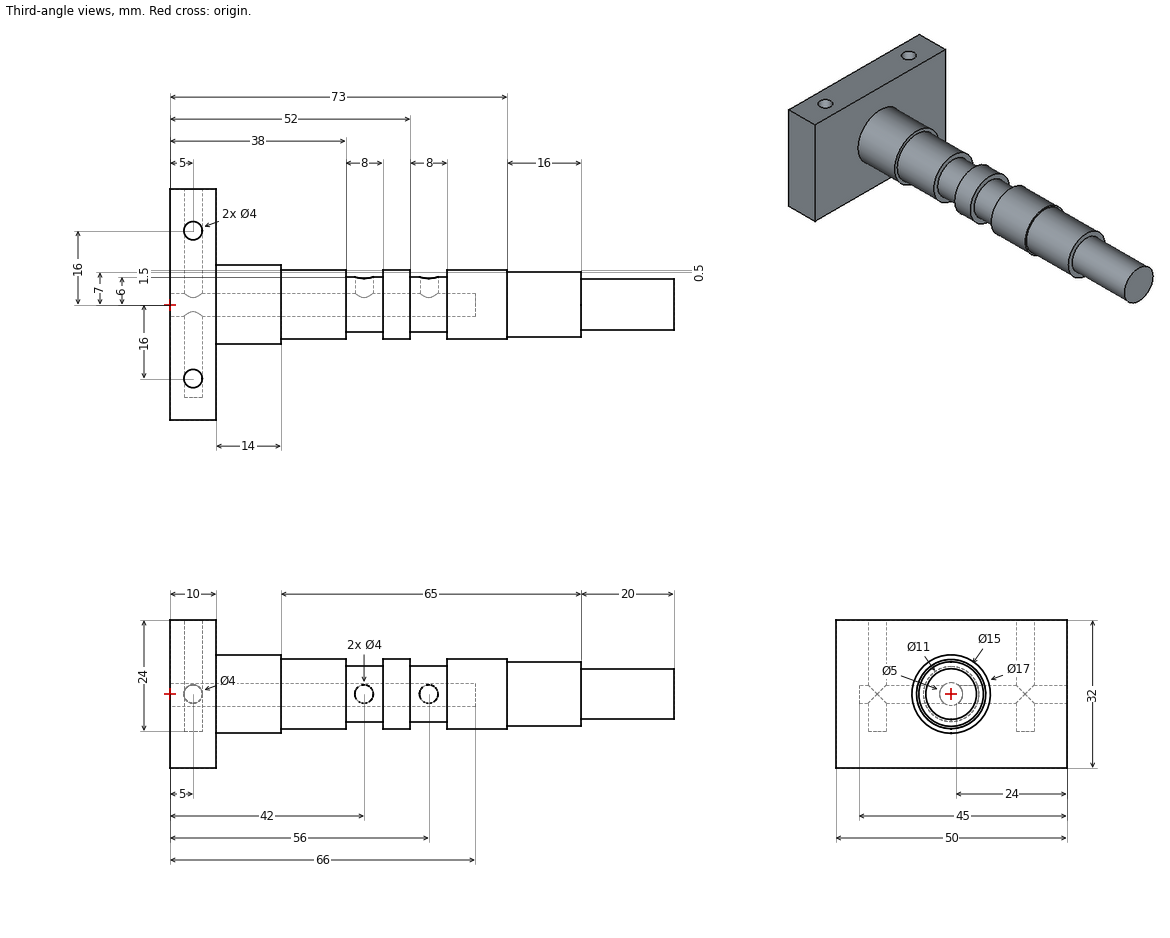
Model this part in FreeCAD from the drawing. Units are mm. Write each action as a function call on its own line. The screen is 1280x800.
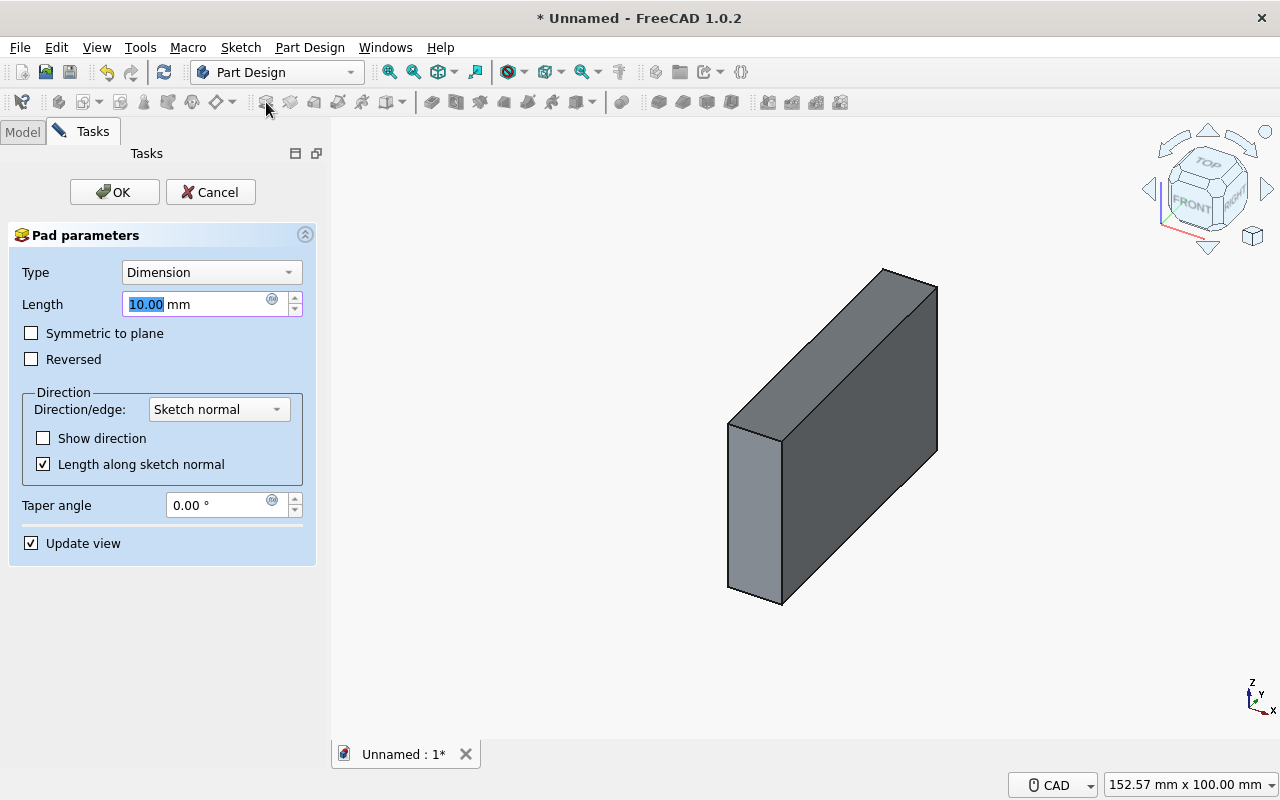
text(10)
key(Tab)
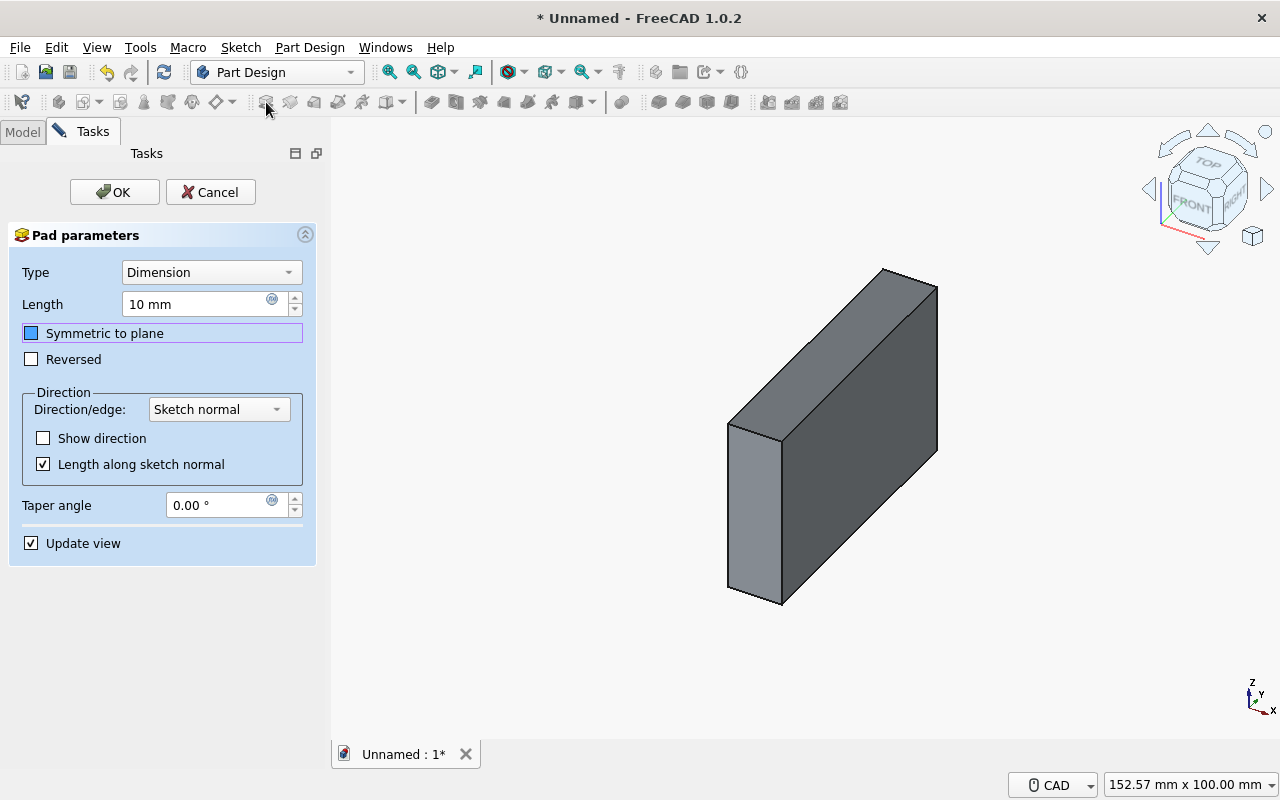
click(115, 192)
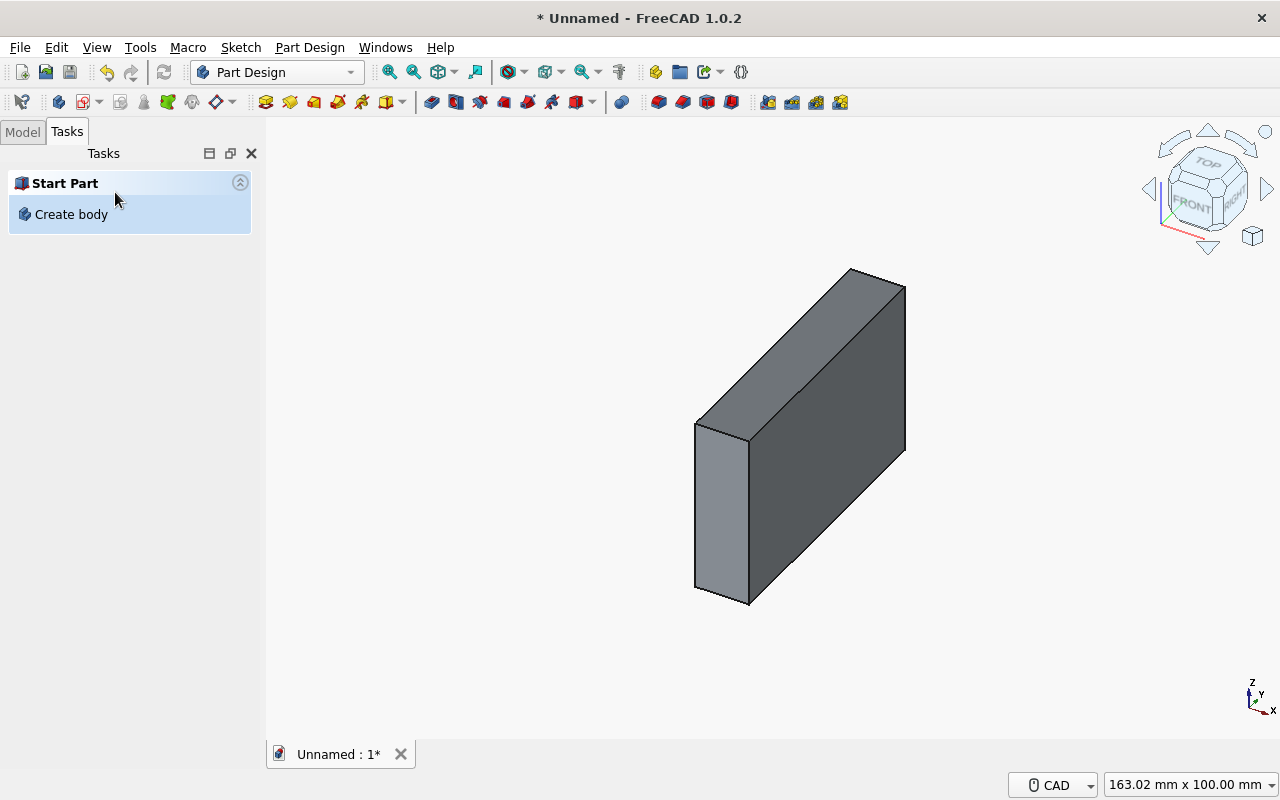
click(849, 423)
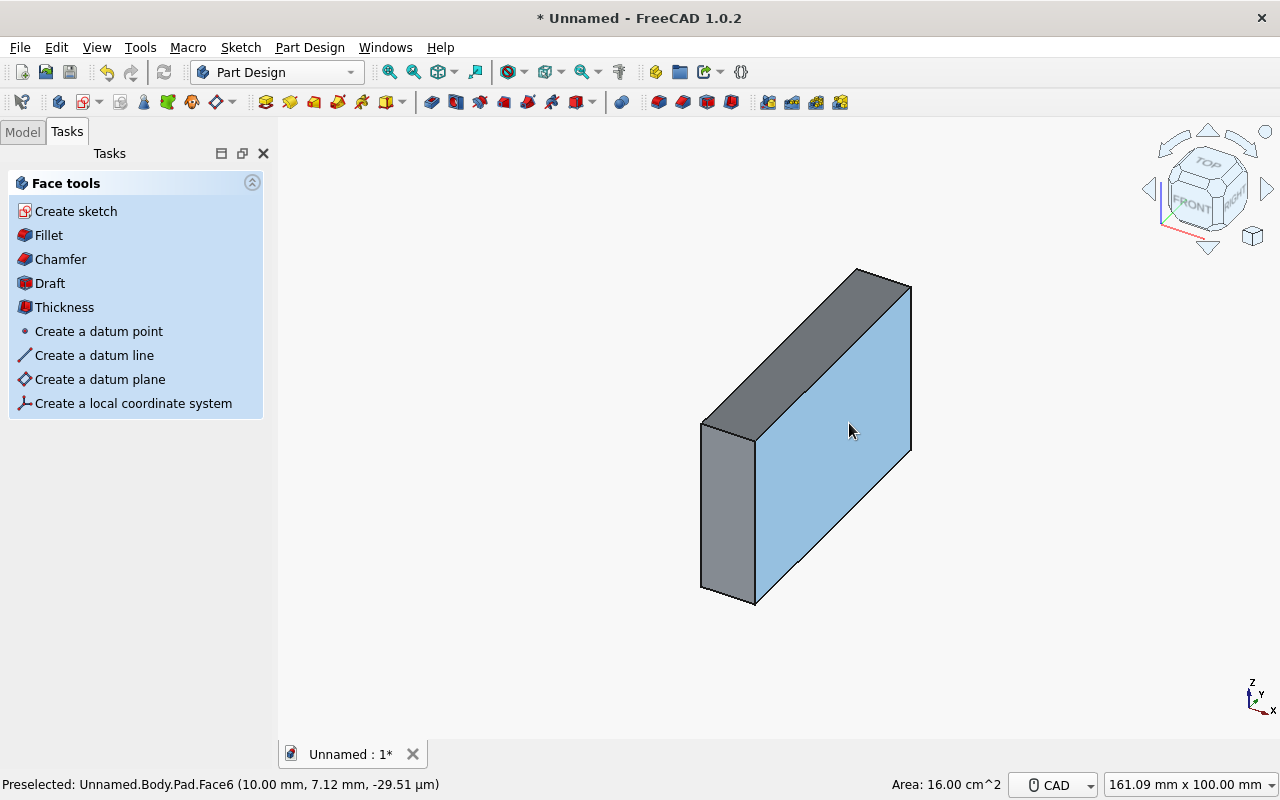
click(84, 102)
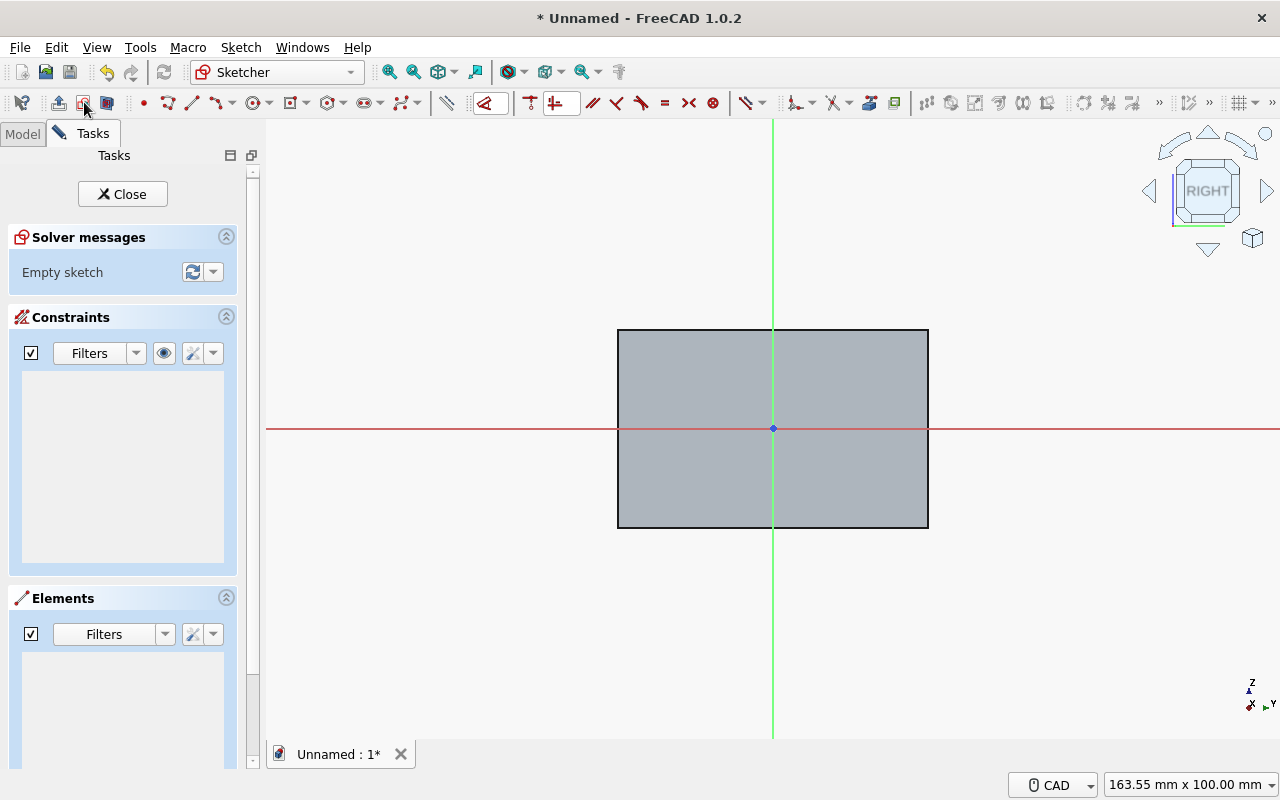
scroll(795, 429, up, 7)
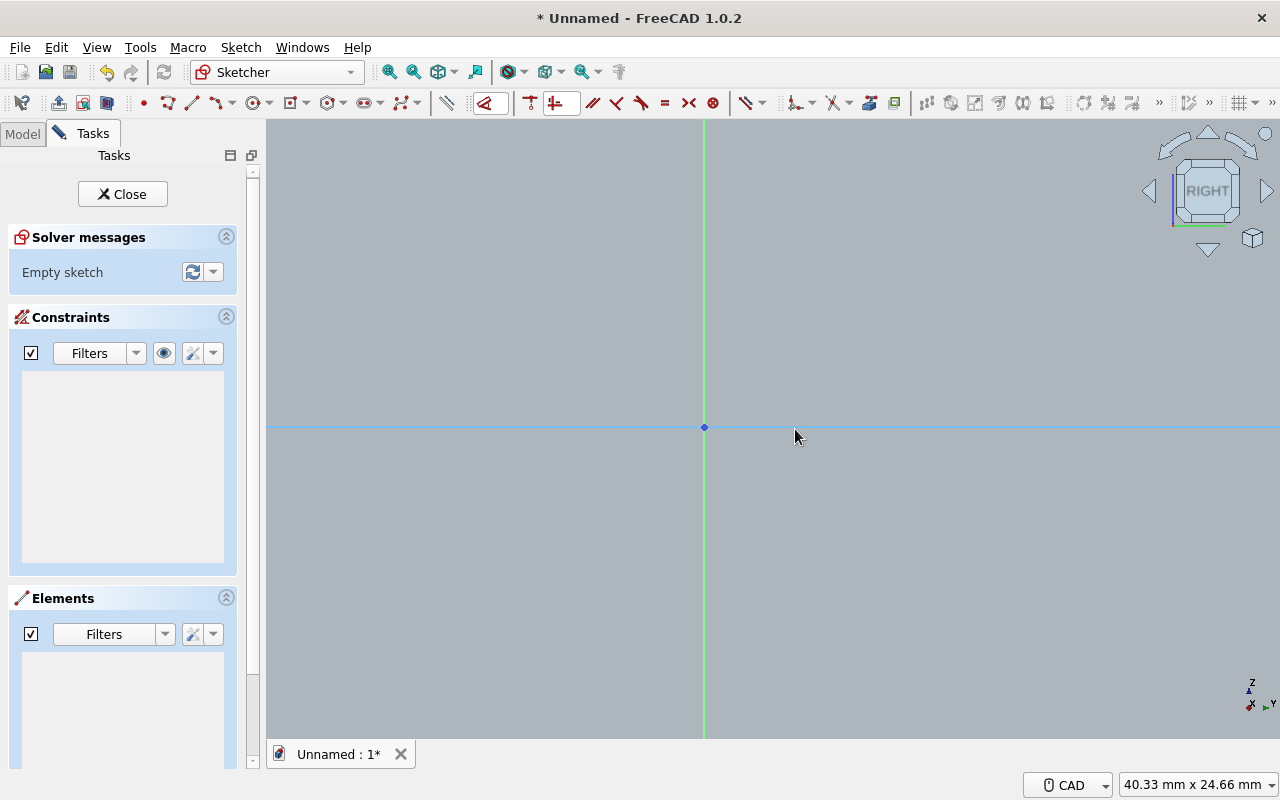
click(254, 104)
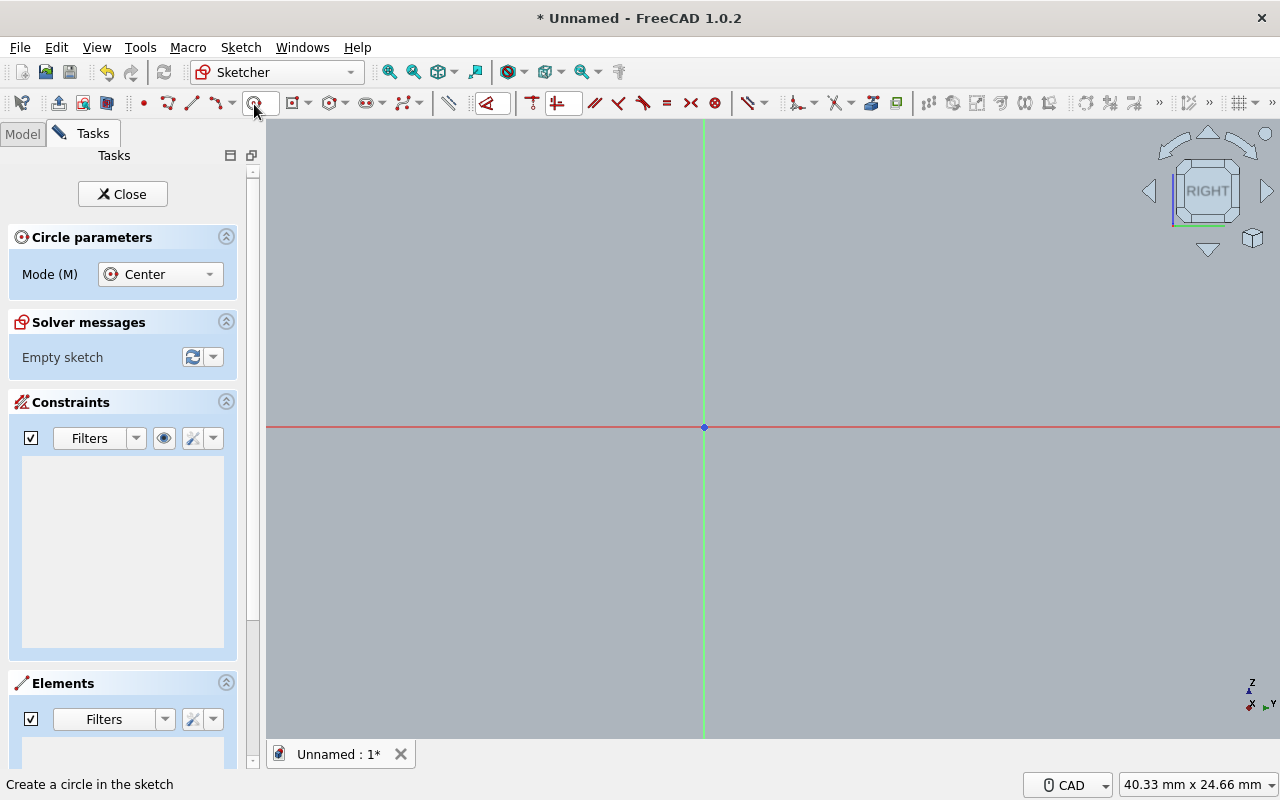
click(704, 427)
move(855, 276)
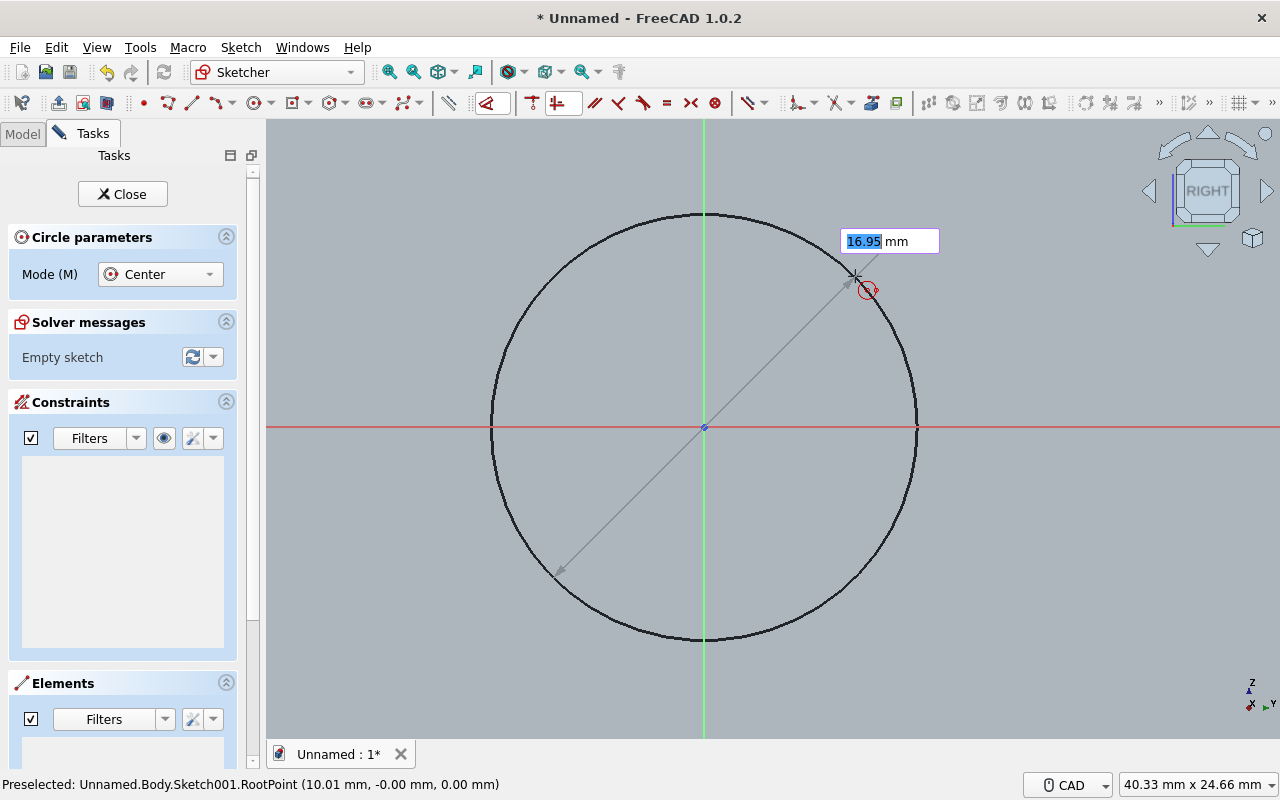
text(17)
key(Return)
key(Escape)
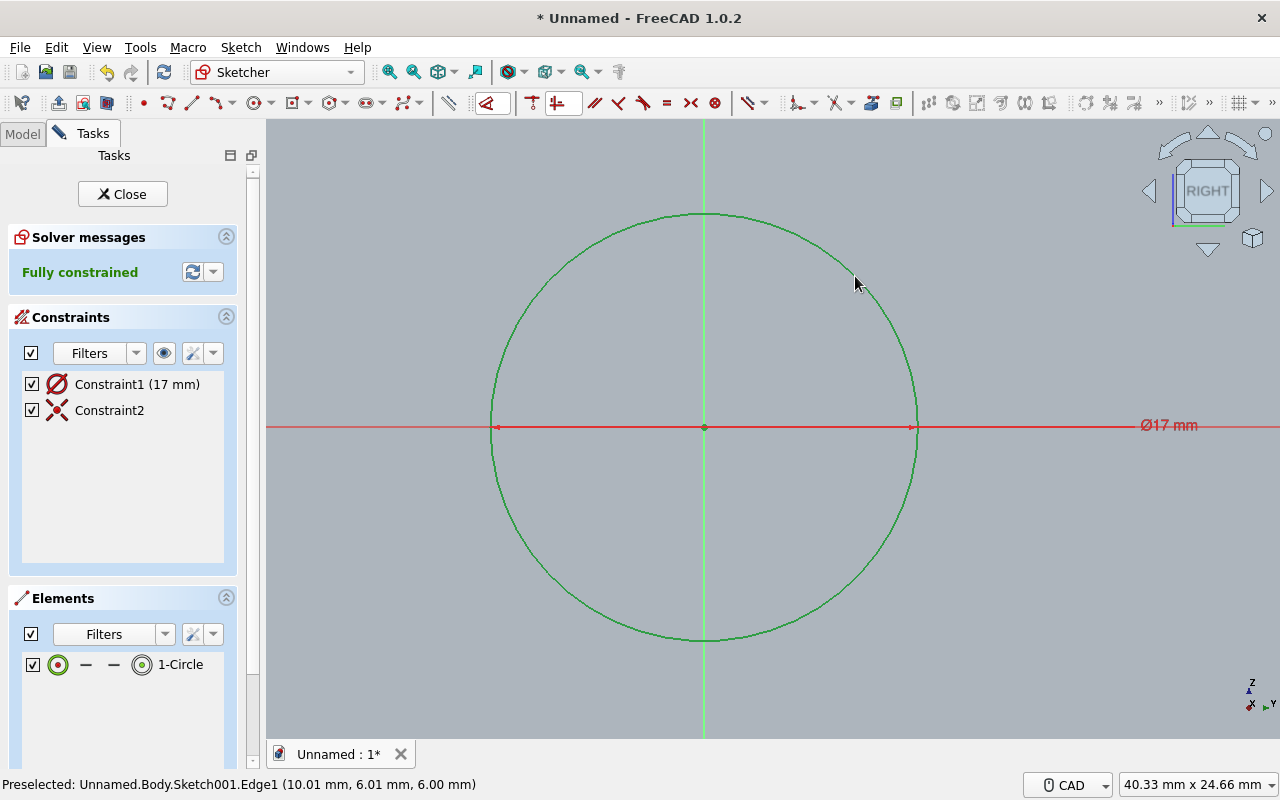
click(123, 194)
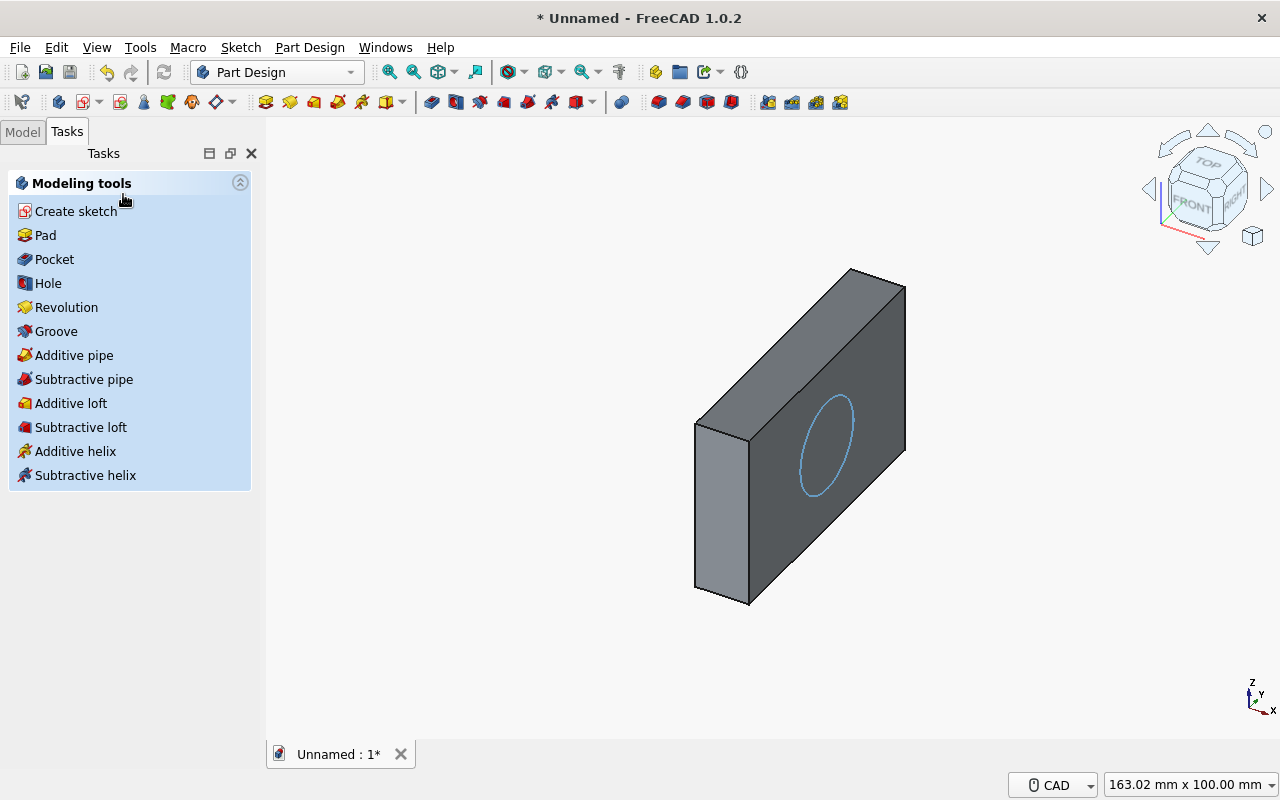
click(266, 102)